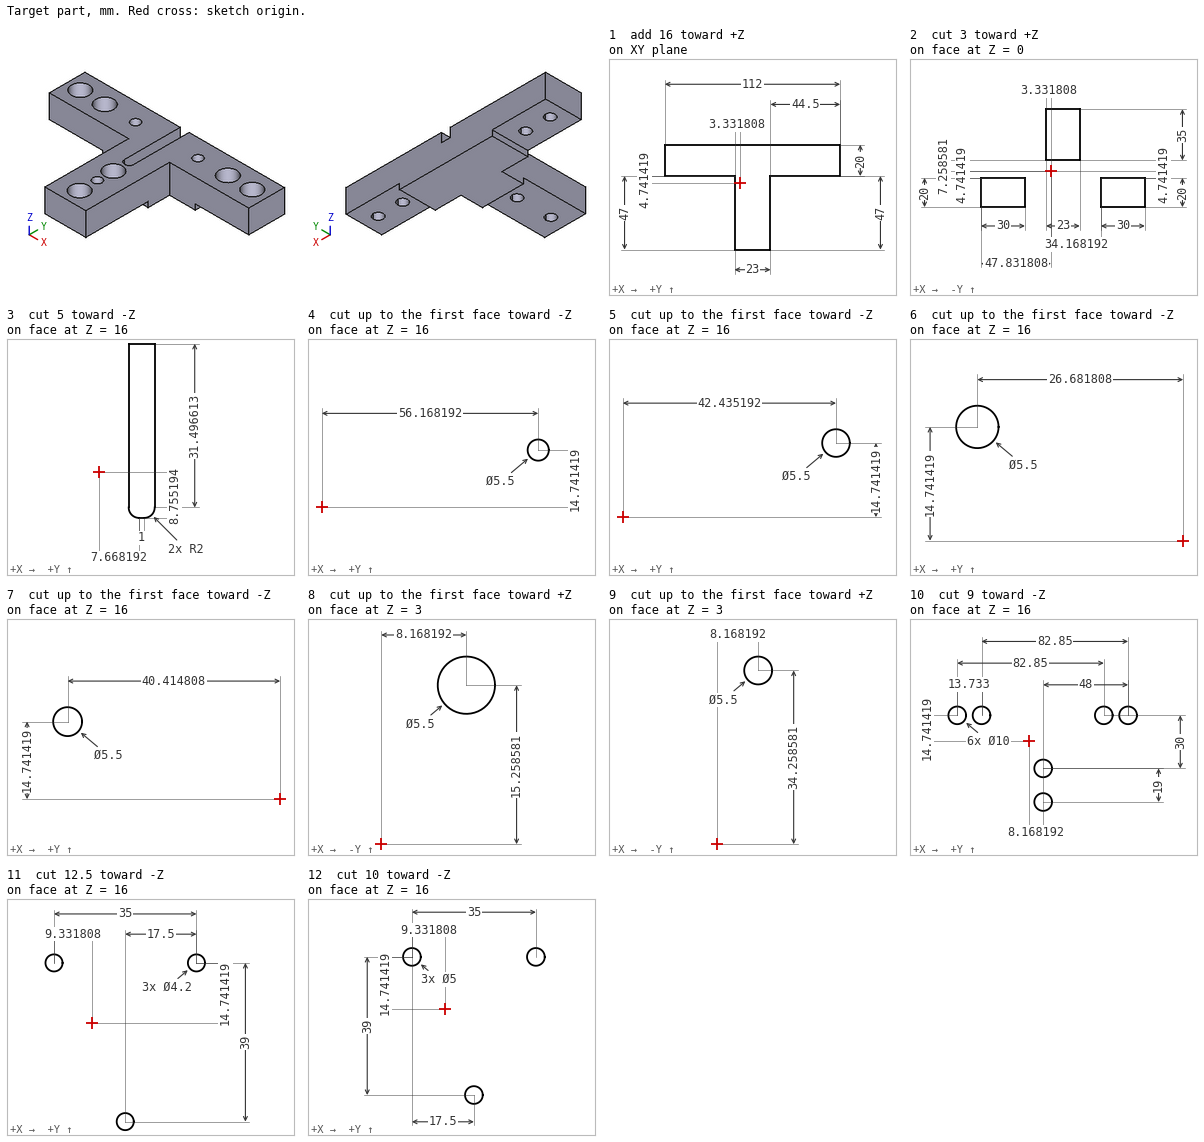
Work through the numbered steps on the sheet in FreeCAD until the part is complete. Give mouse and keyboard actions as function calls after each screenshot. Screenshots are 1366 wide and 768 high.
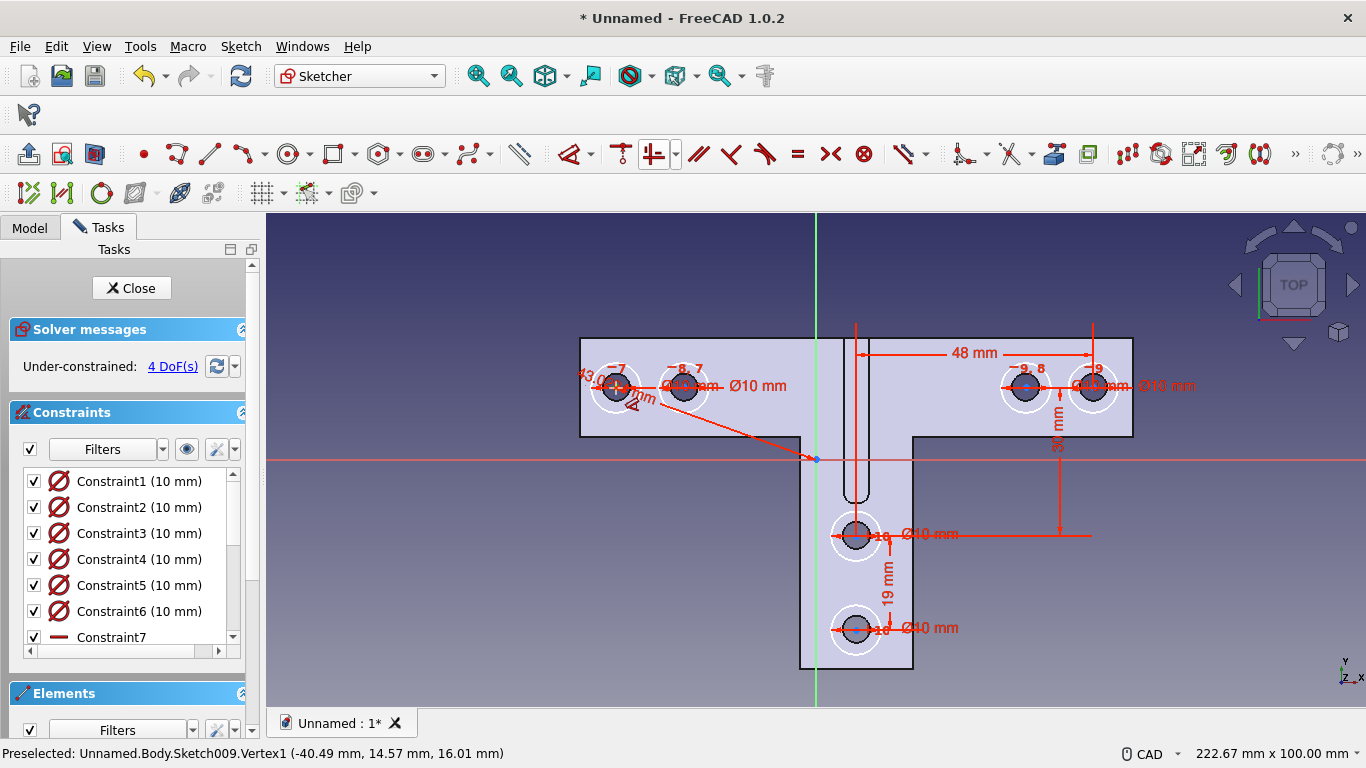
click(1026, 388)
click(727, 354)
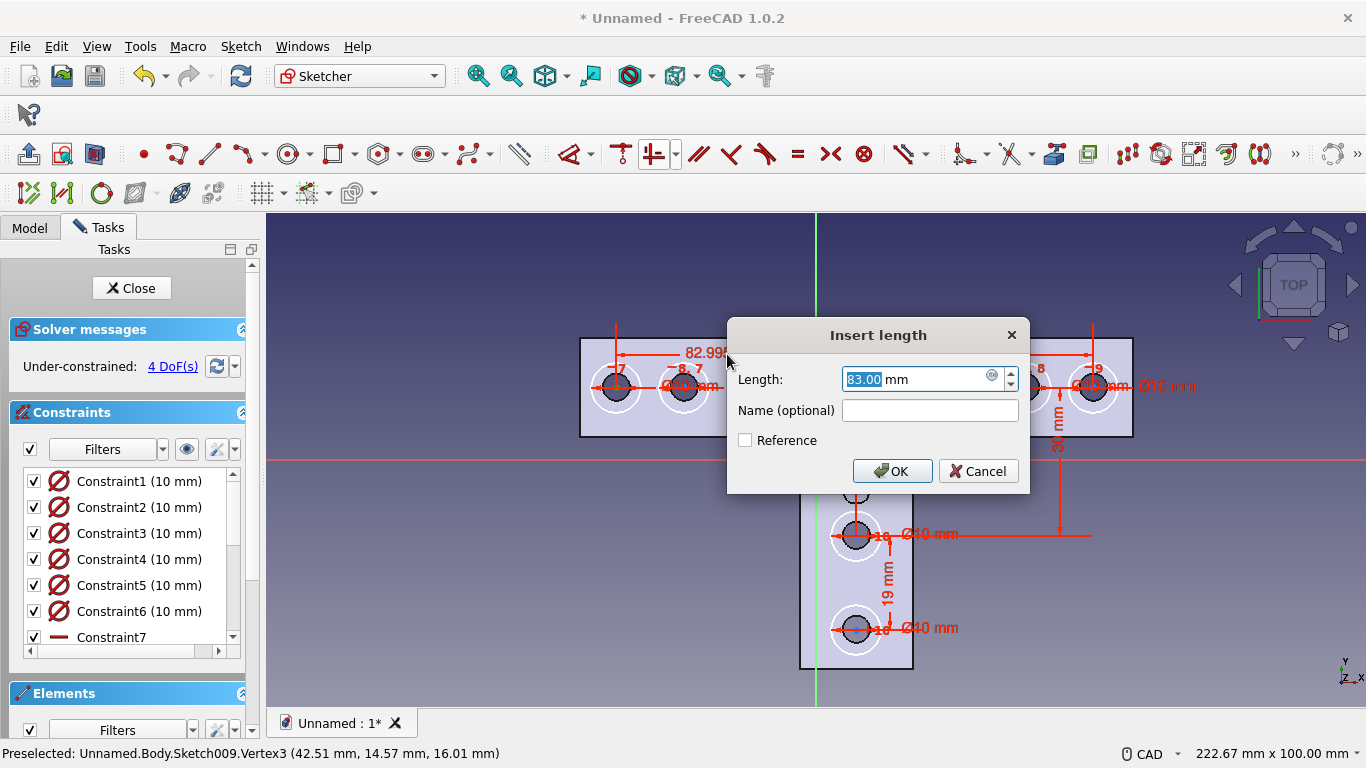
text(82.85)
key(Return)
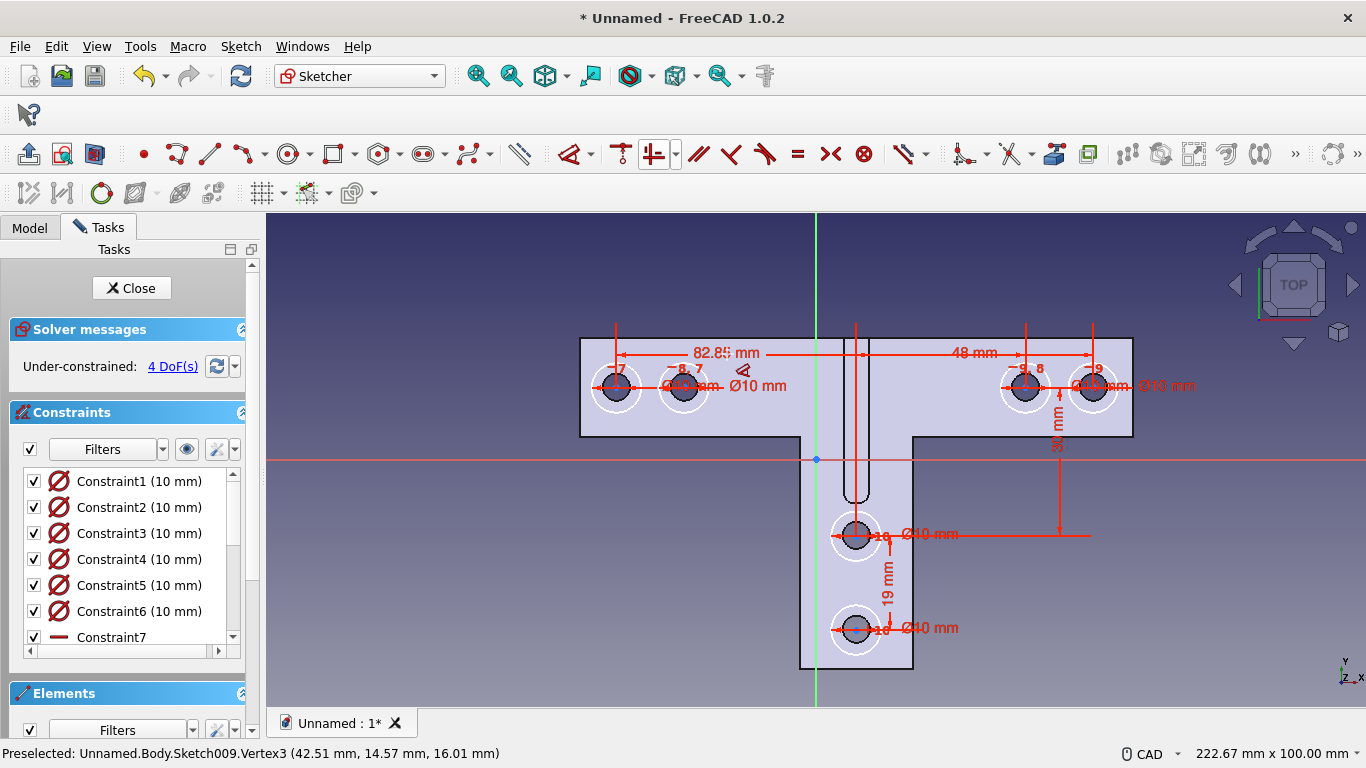
click(684, 388)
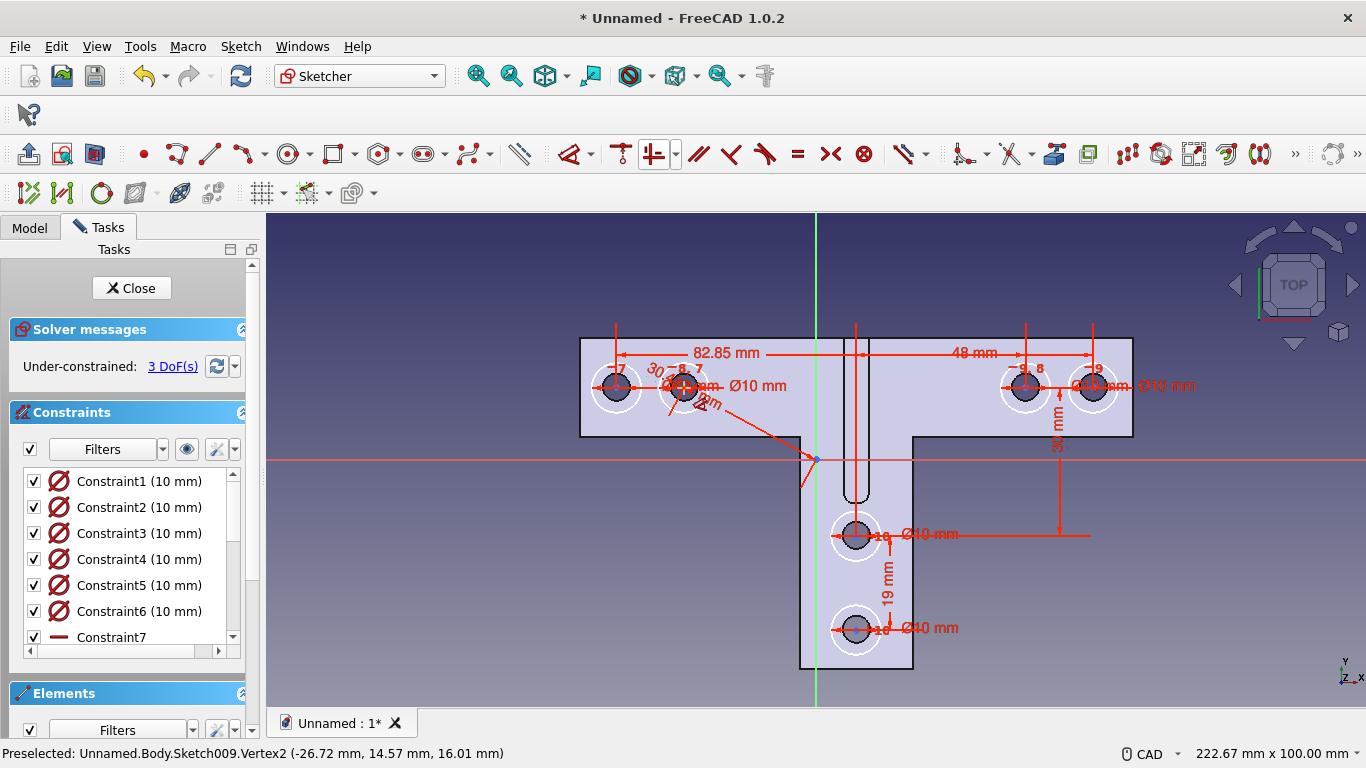
click(1093, 388)
click(889, 354)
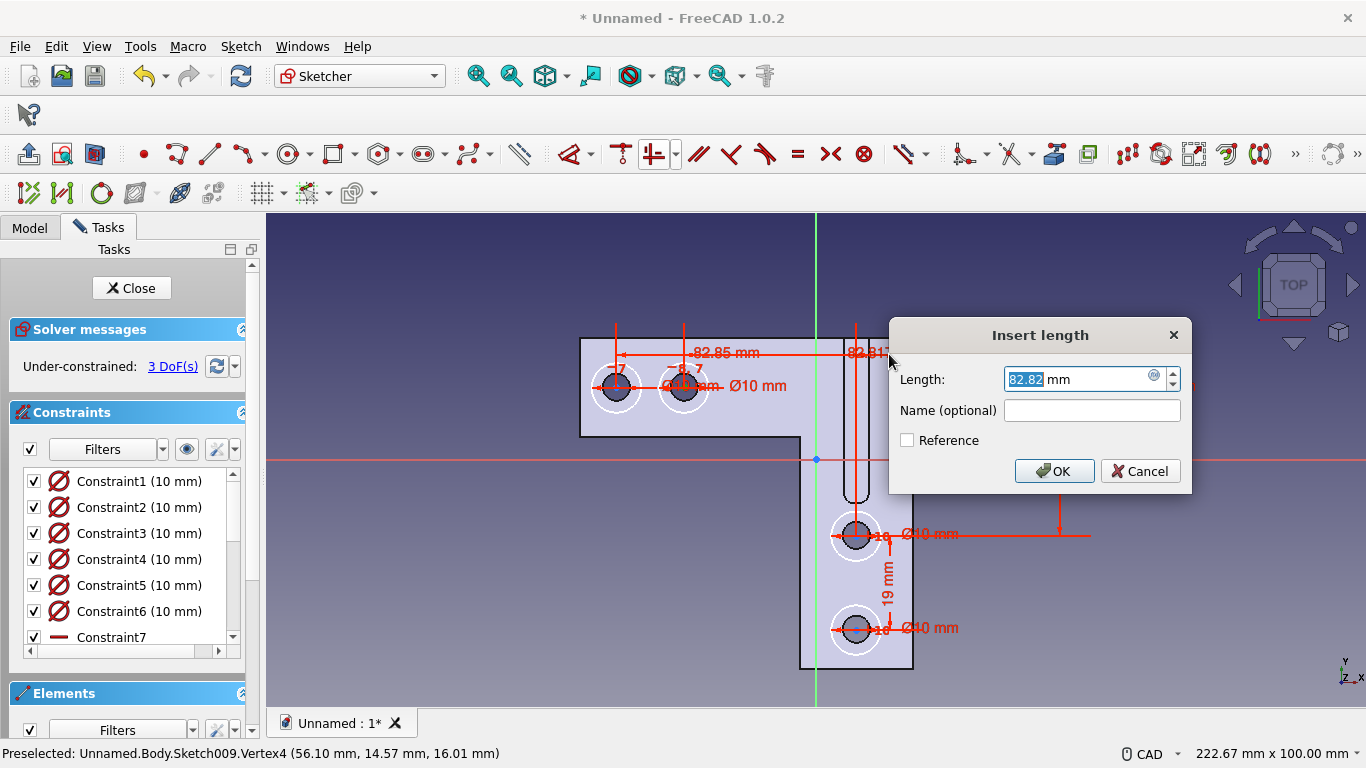
text(82.85)
key(Return)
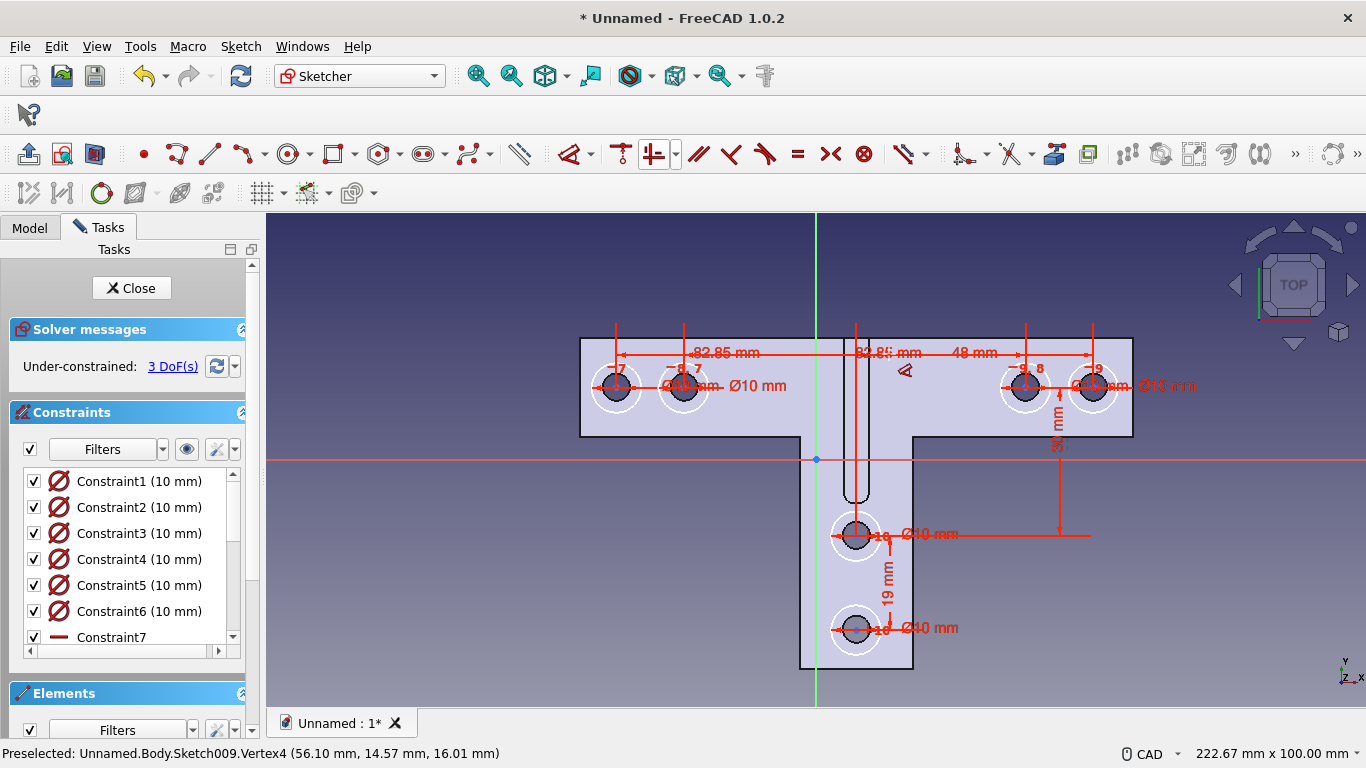
click(616, 388)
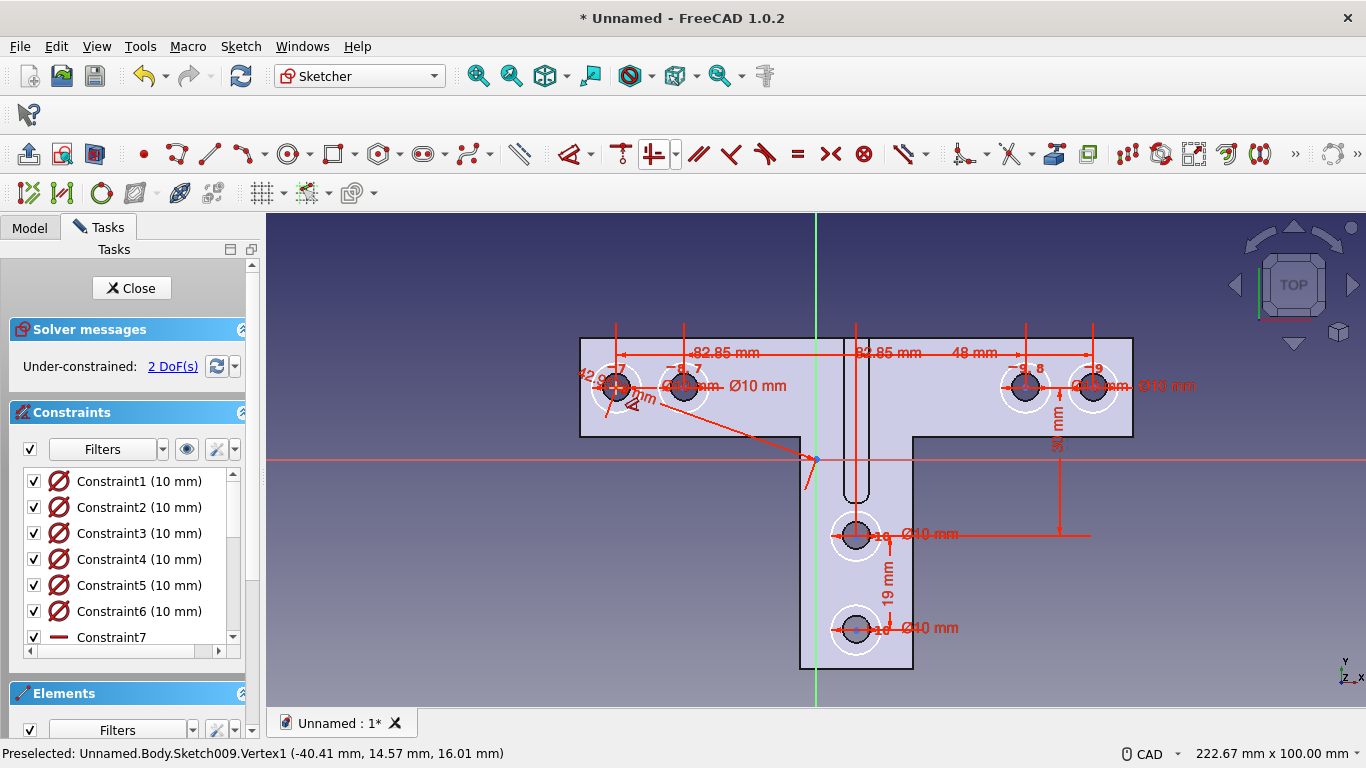
click(684, 388)
click(650, 354)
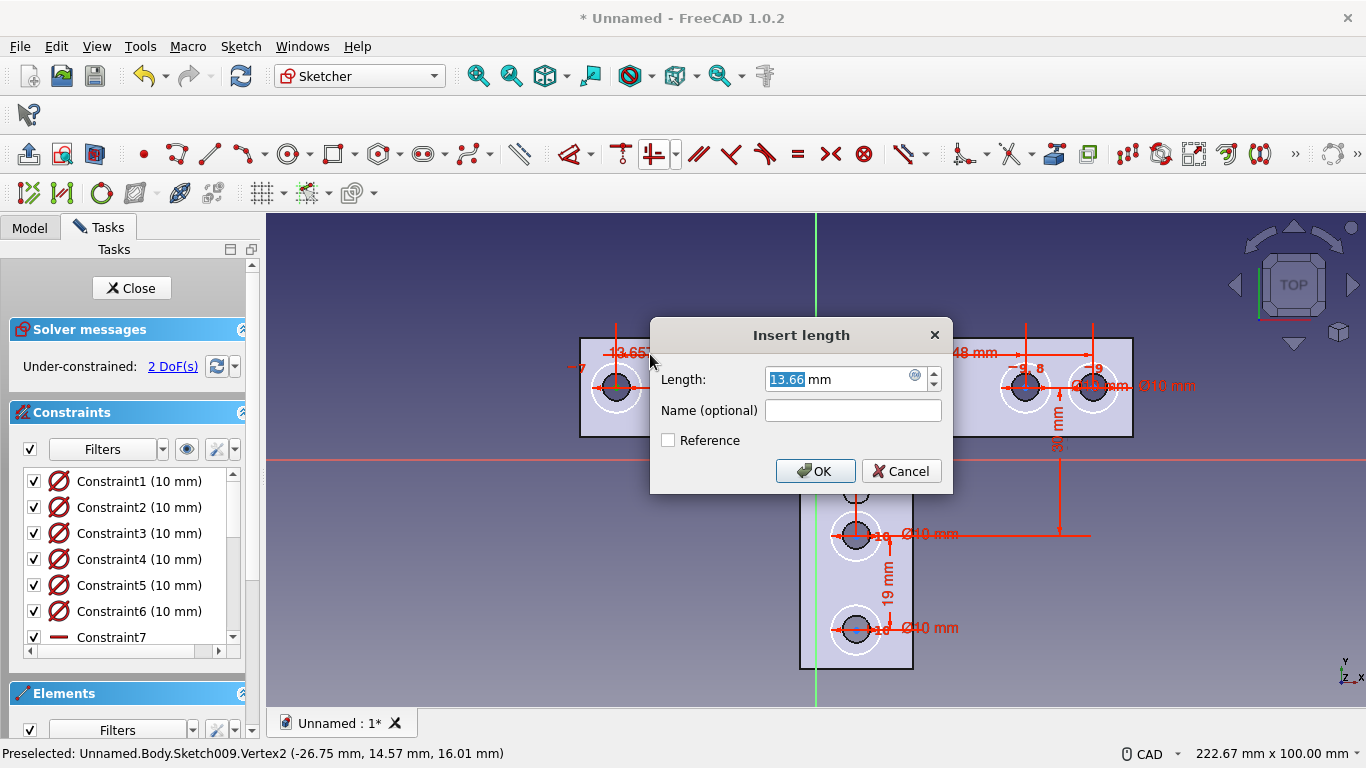
text(13.733)
key(Return)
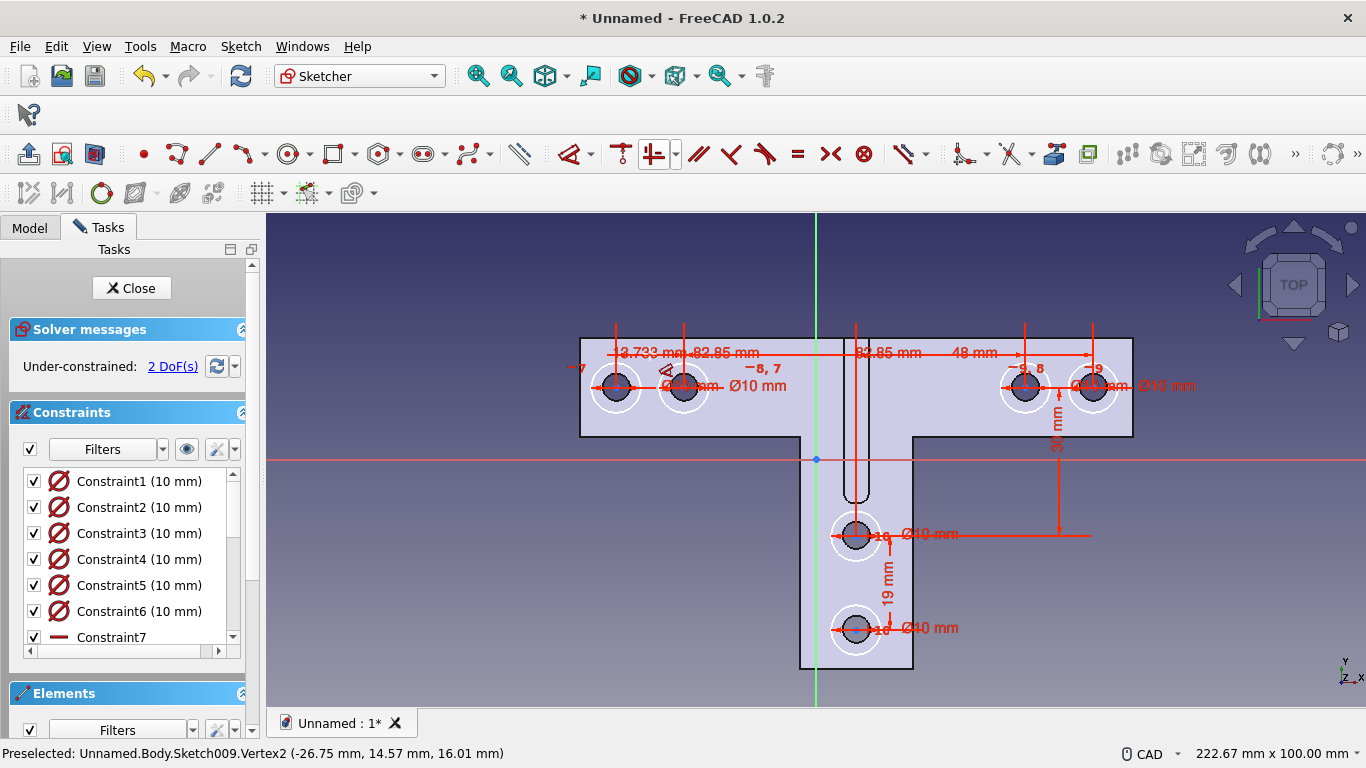
click(856, 536)
click(836, 426)